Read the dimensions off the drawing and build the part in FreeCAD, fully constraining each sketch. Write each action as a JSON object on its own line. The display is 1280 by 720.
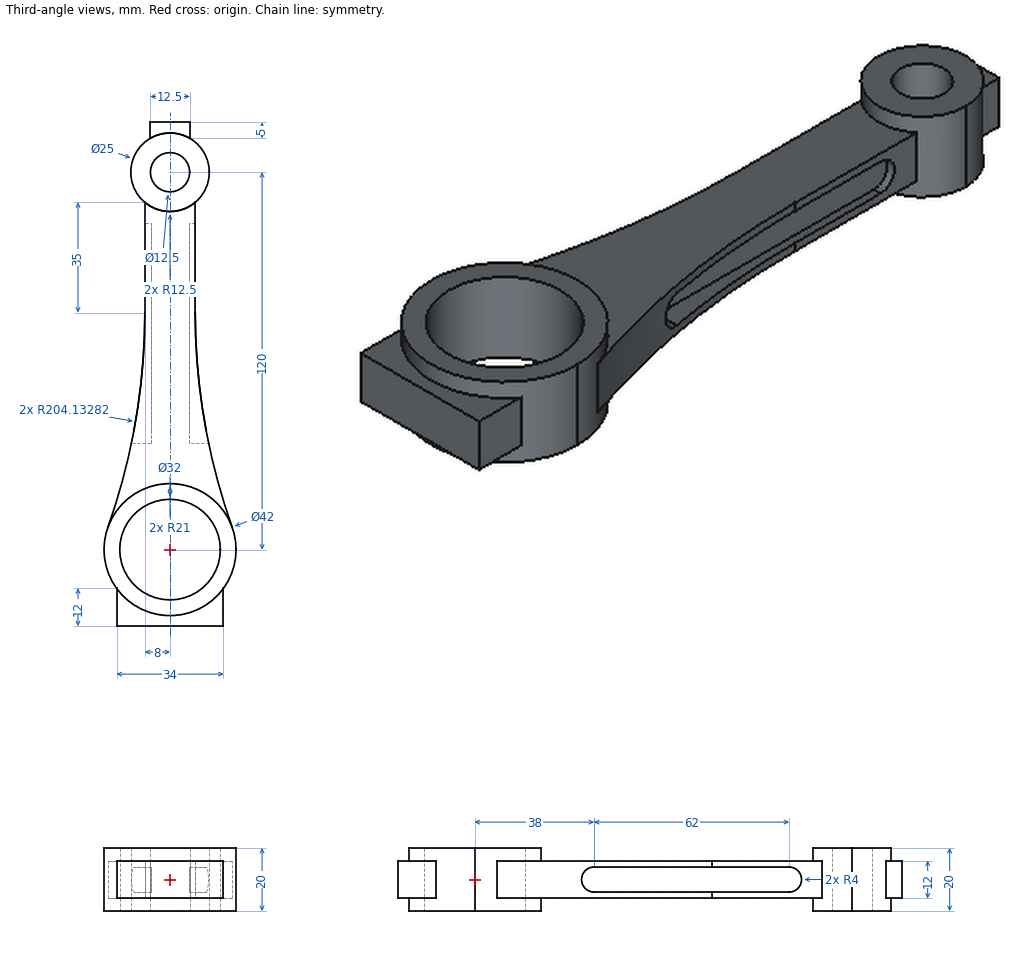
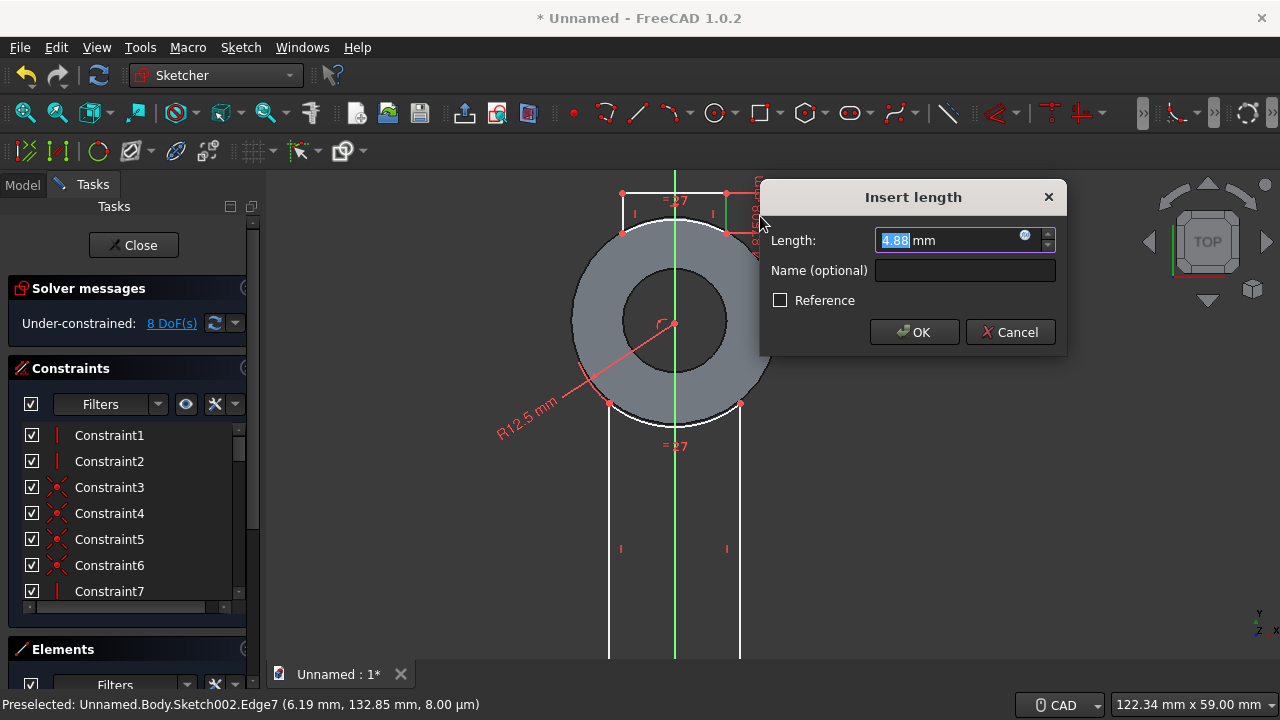
{"action": "type", "text": "5"}
{"action": "key", "text": "Return"}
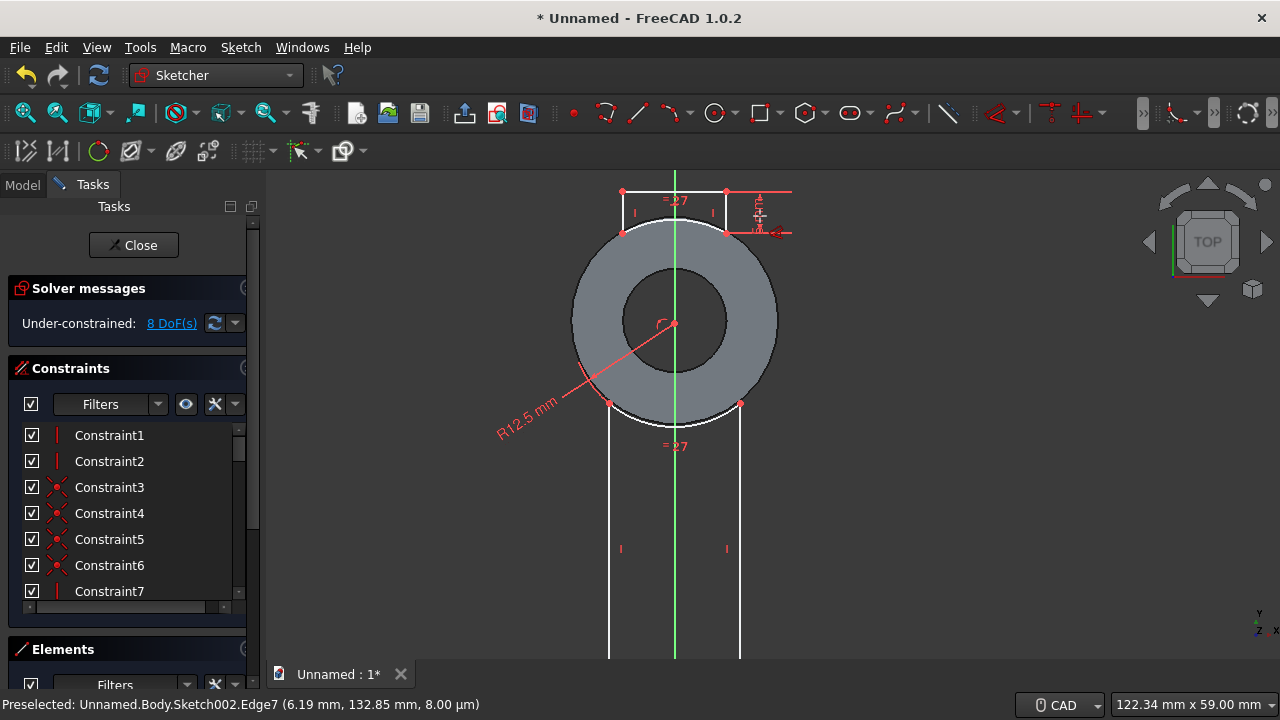
{"action": "left_click", "coordinate": [623, 205]}
{"action": "left_click", "coordinate": [589, 216]}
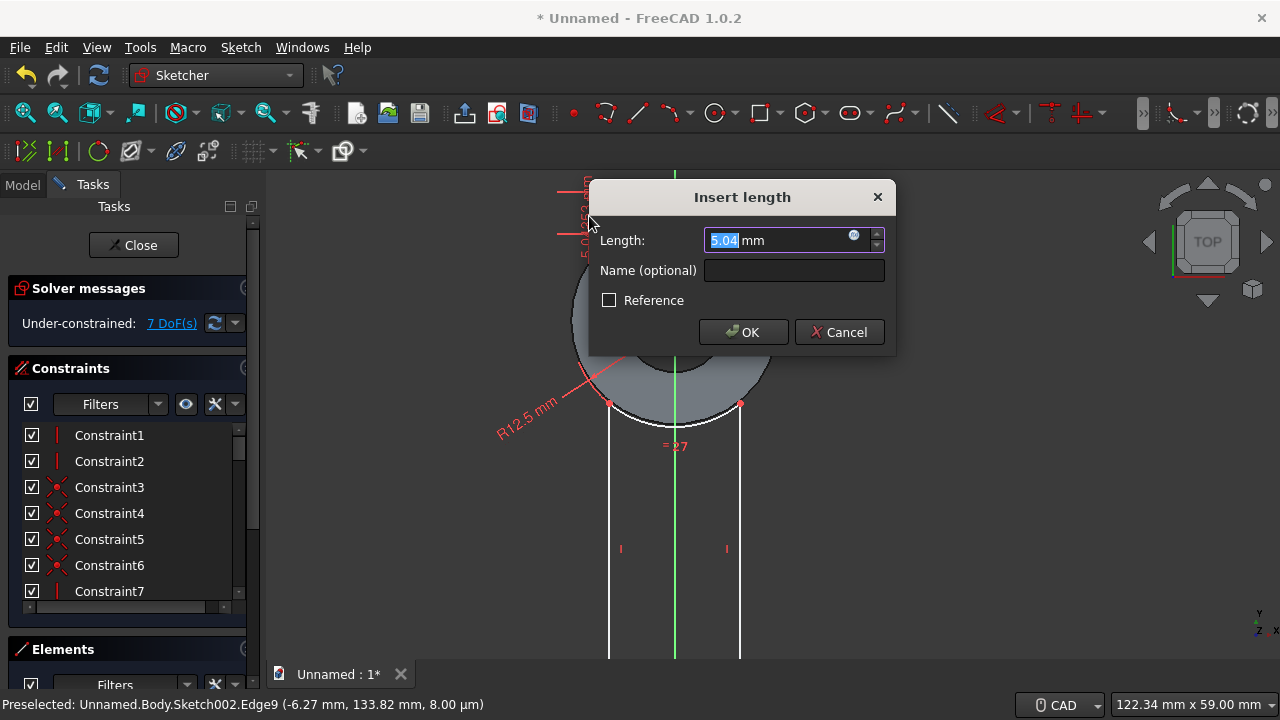
{"action": "type", "text": "5"}
{"action": "key", "text": "Return"}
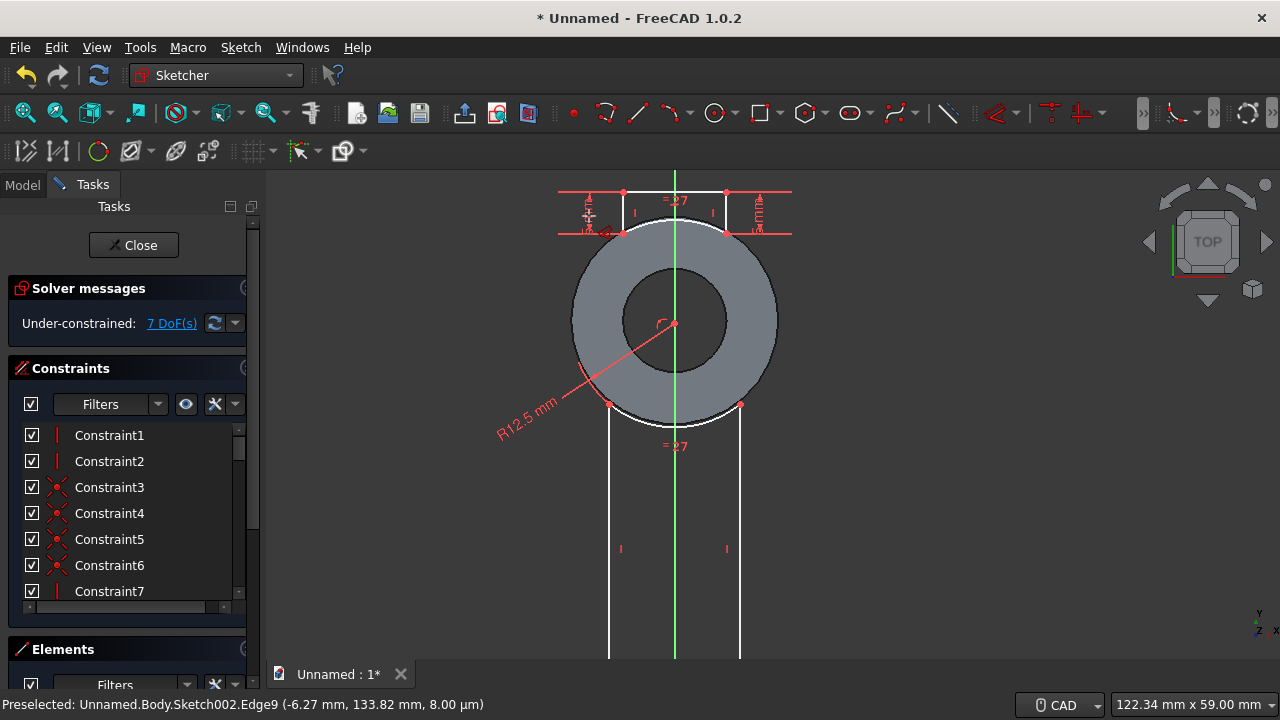
{"action": "scroll", "coordinate": [714, 271], "scroll_direction": "down", "scroll_amount": 7}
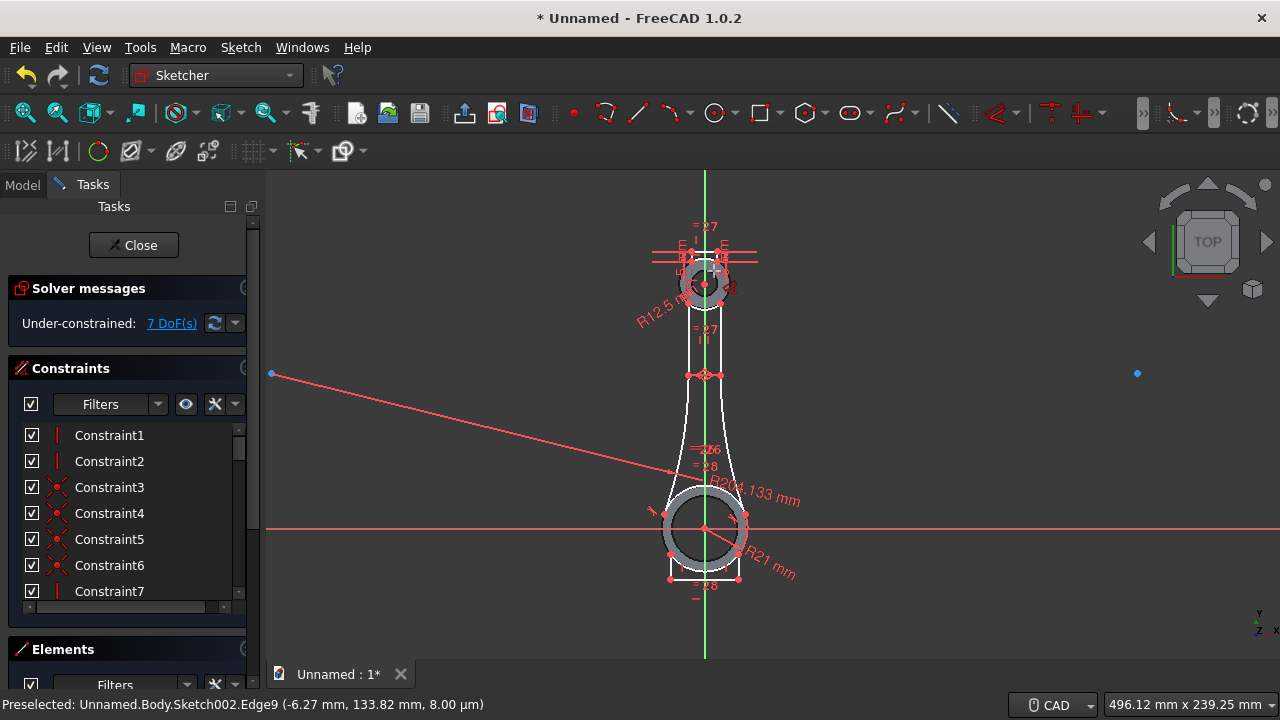
{"action": "left_click", "coordinate": [689, 325]}
{"action": "left_click", "coordinate": [655, 340]}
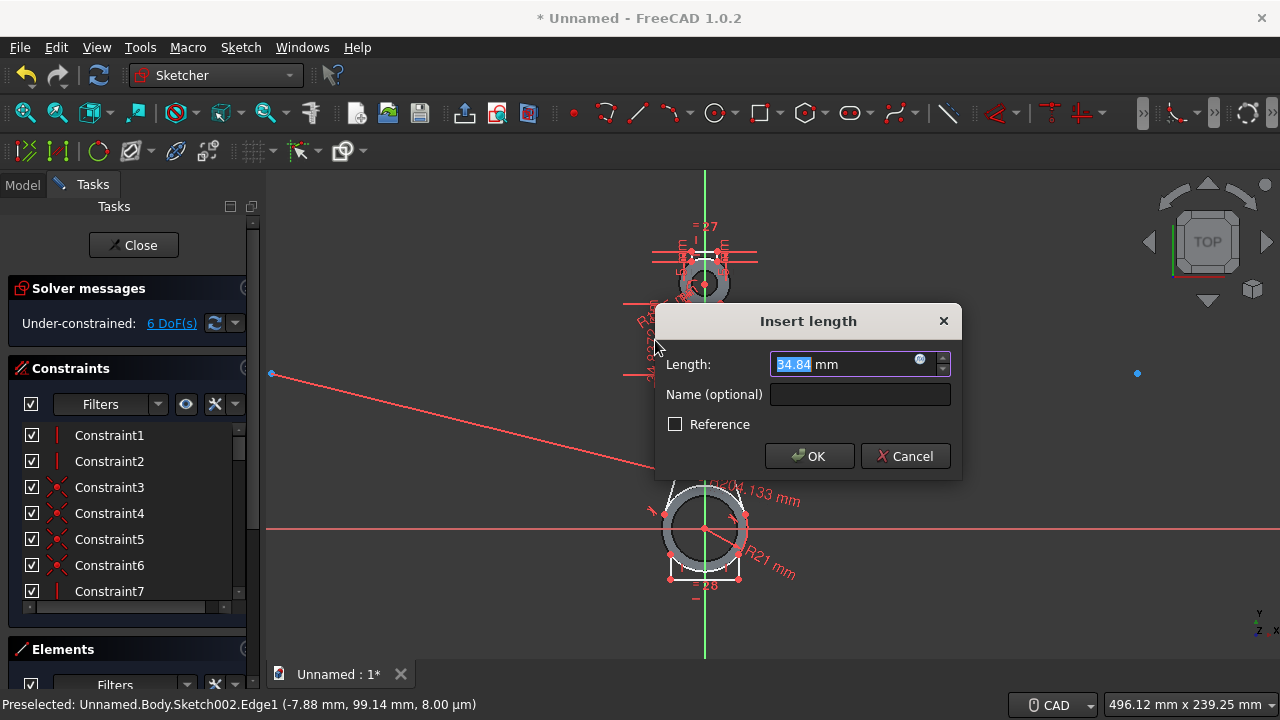
{"action": "type", "text": "35"}
{"action": "key", "text": "Return"}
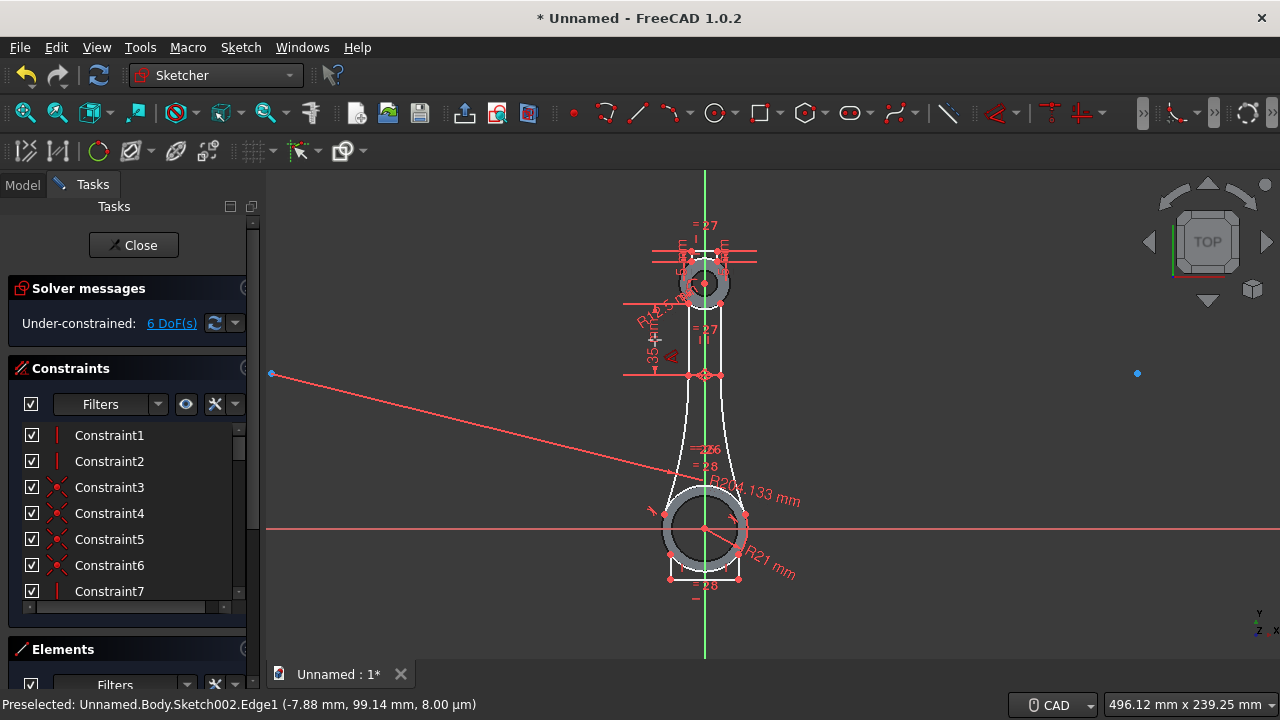
{"action": "scroll", "coordinate": [671, 570], "scroll_direction": "up", "scroll_amount": 3}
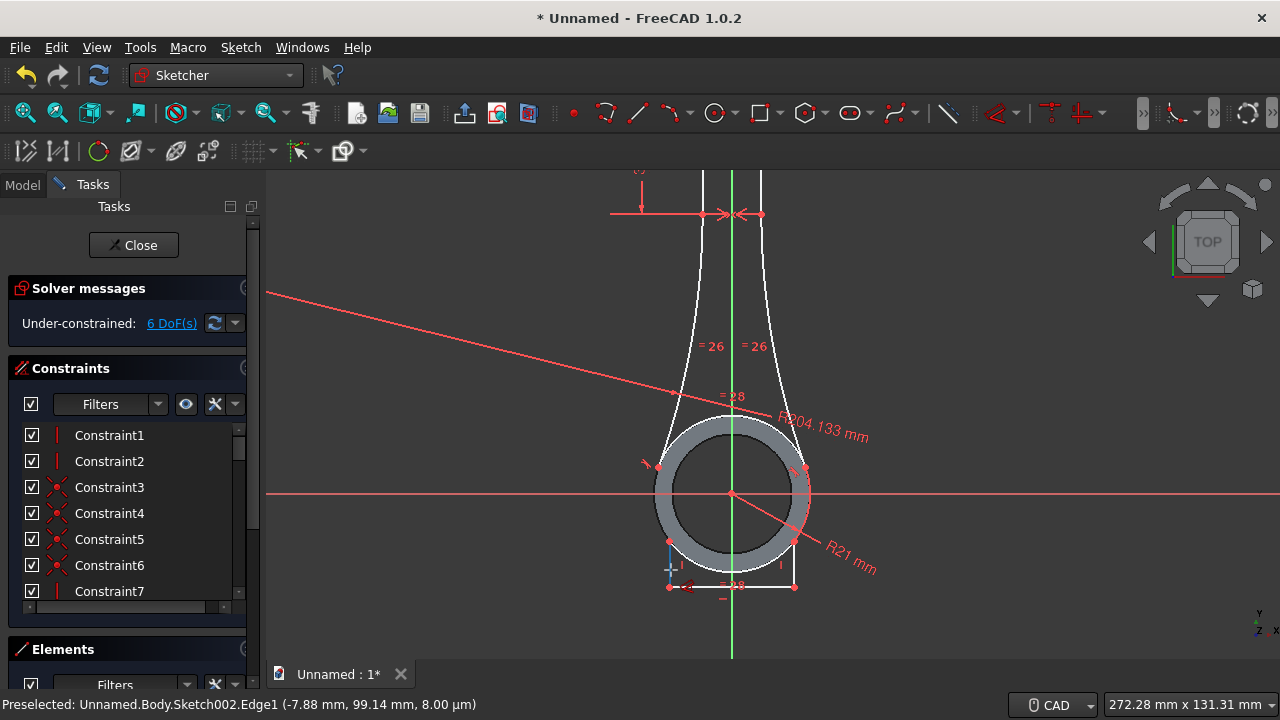
{"action": "left_click", "coordinate": [670, 569]}
{"action": "left_click", "coordinate": [636, 564]}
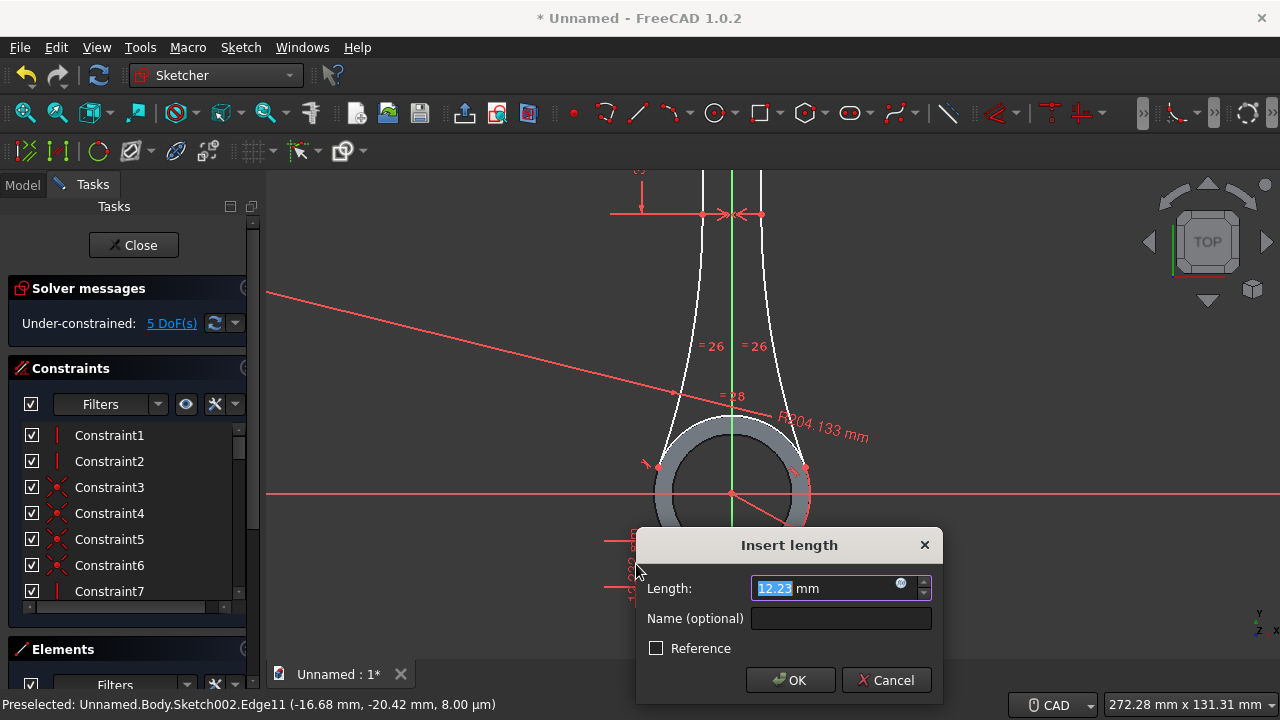
{"action": "type", "text": "12"}
{"action": "key", "text": "Return"}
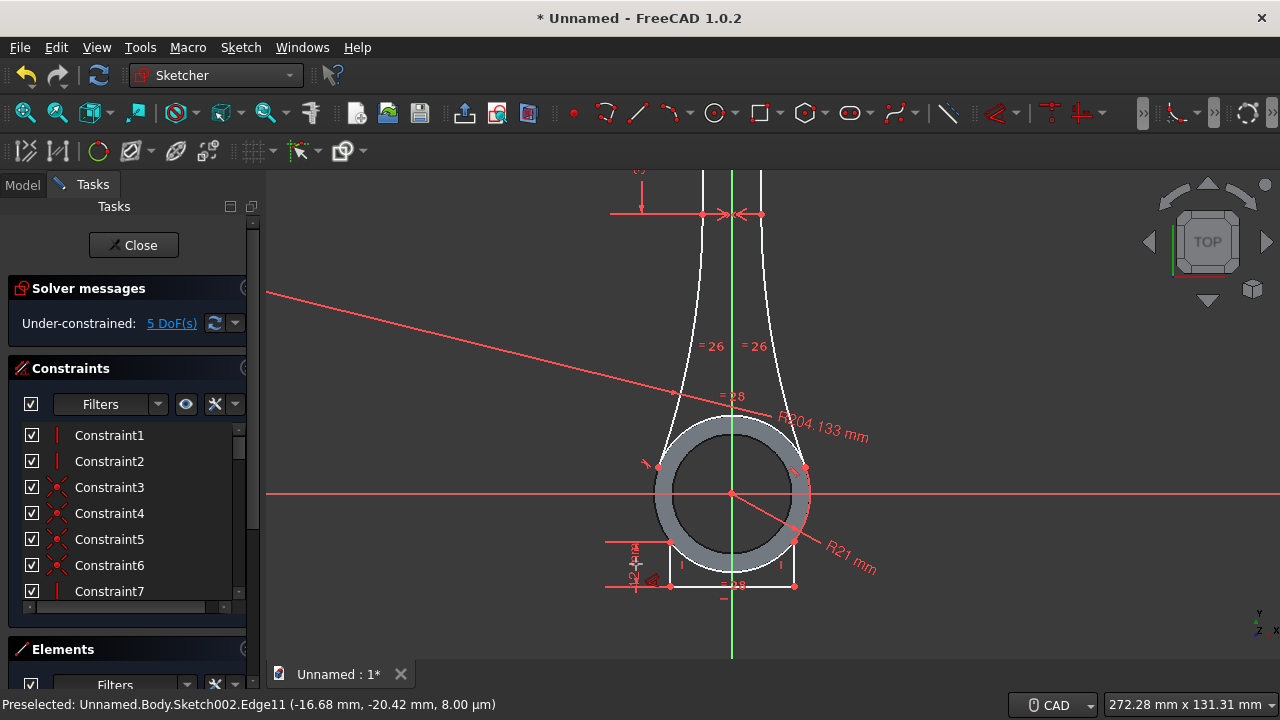
{"action": "left_click", "coordinate": [707, 587]}
{"action": "left_click", "coordinate": [704, 621]}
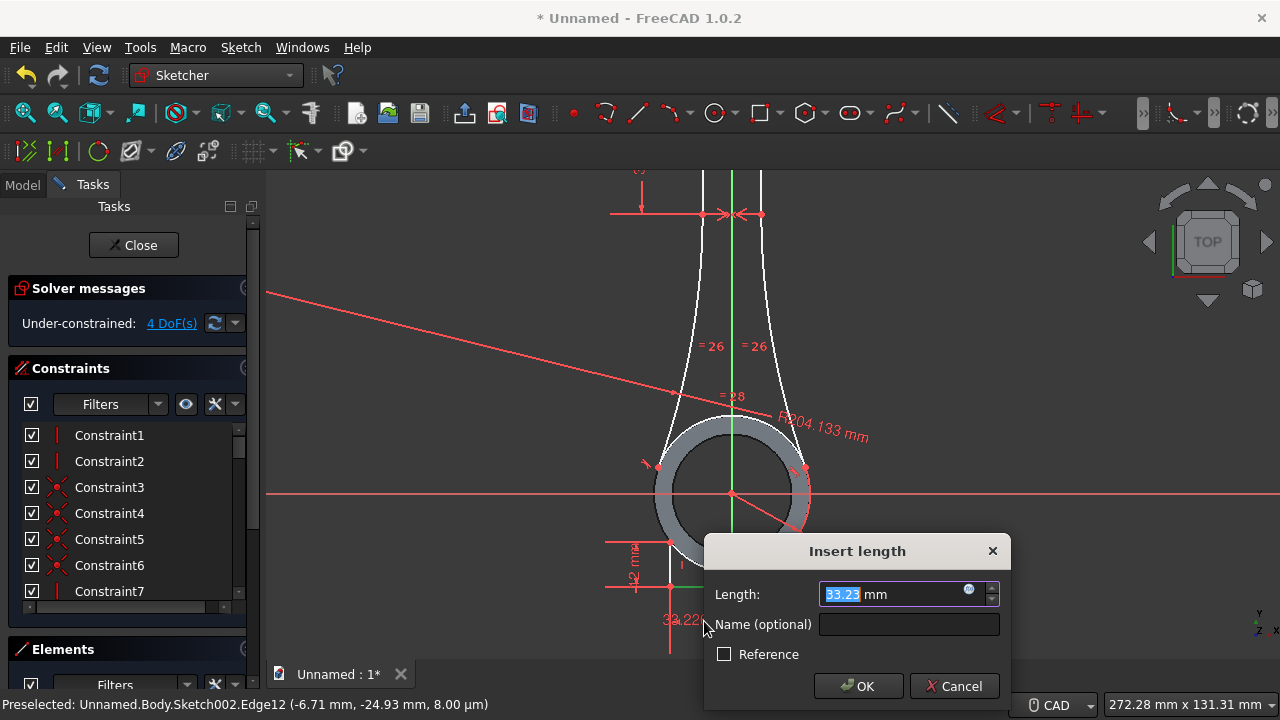
{"action": "type", "text": "34"}
{"action": "key", "text": "Return"}